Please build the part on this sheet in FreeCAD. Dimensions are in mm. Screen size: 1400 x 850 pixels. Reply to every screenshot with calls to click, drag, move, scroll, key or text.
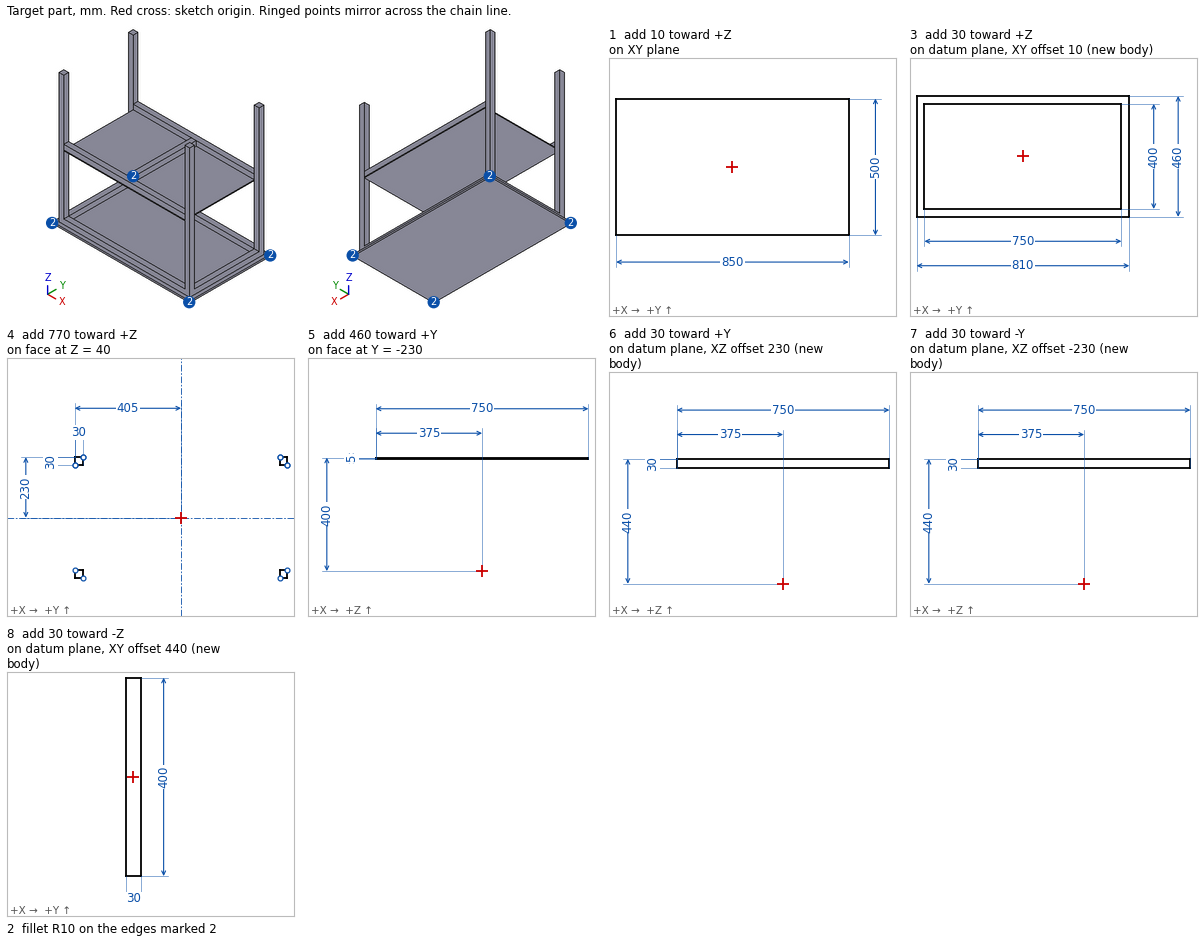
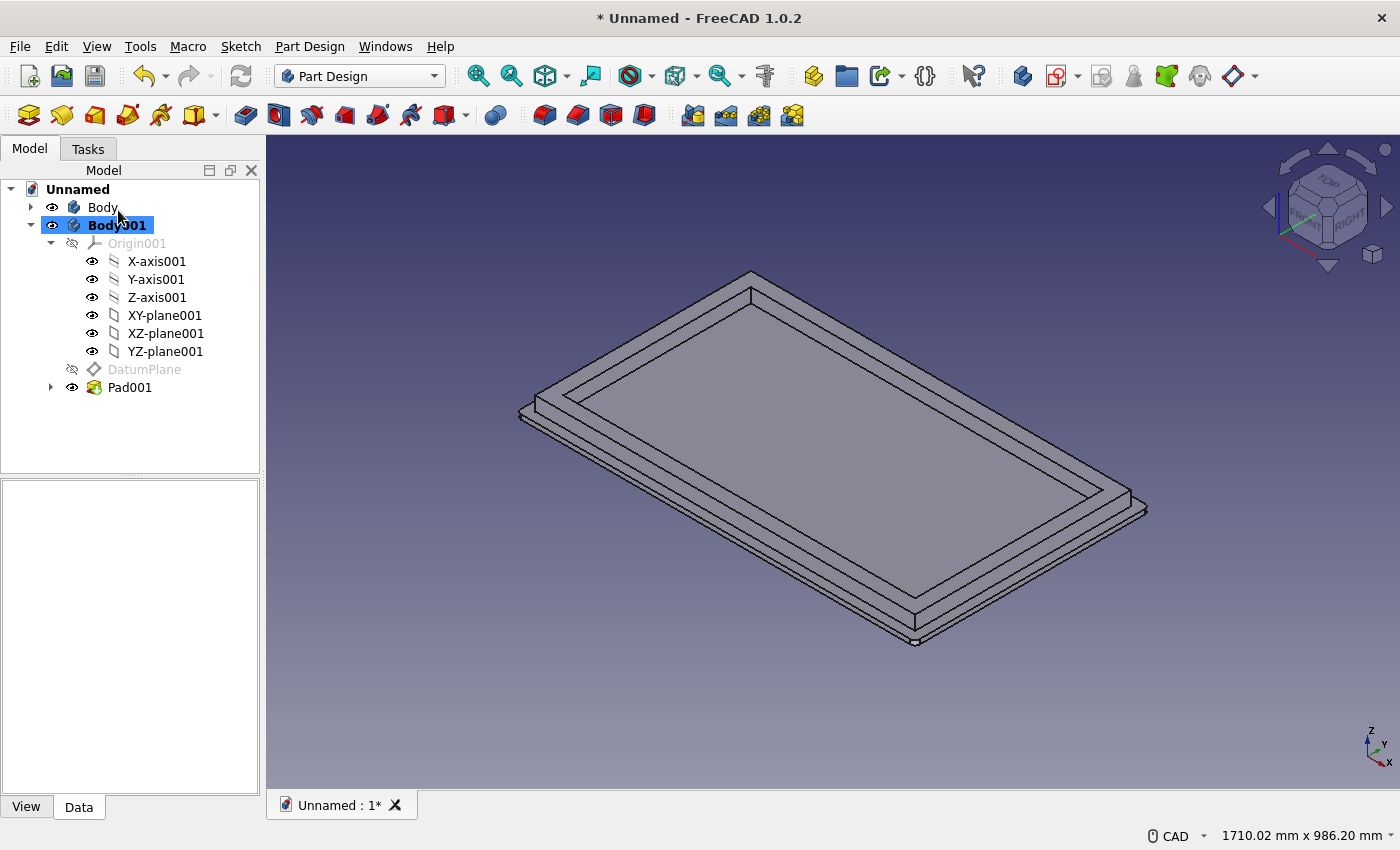
click(1049, 525)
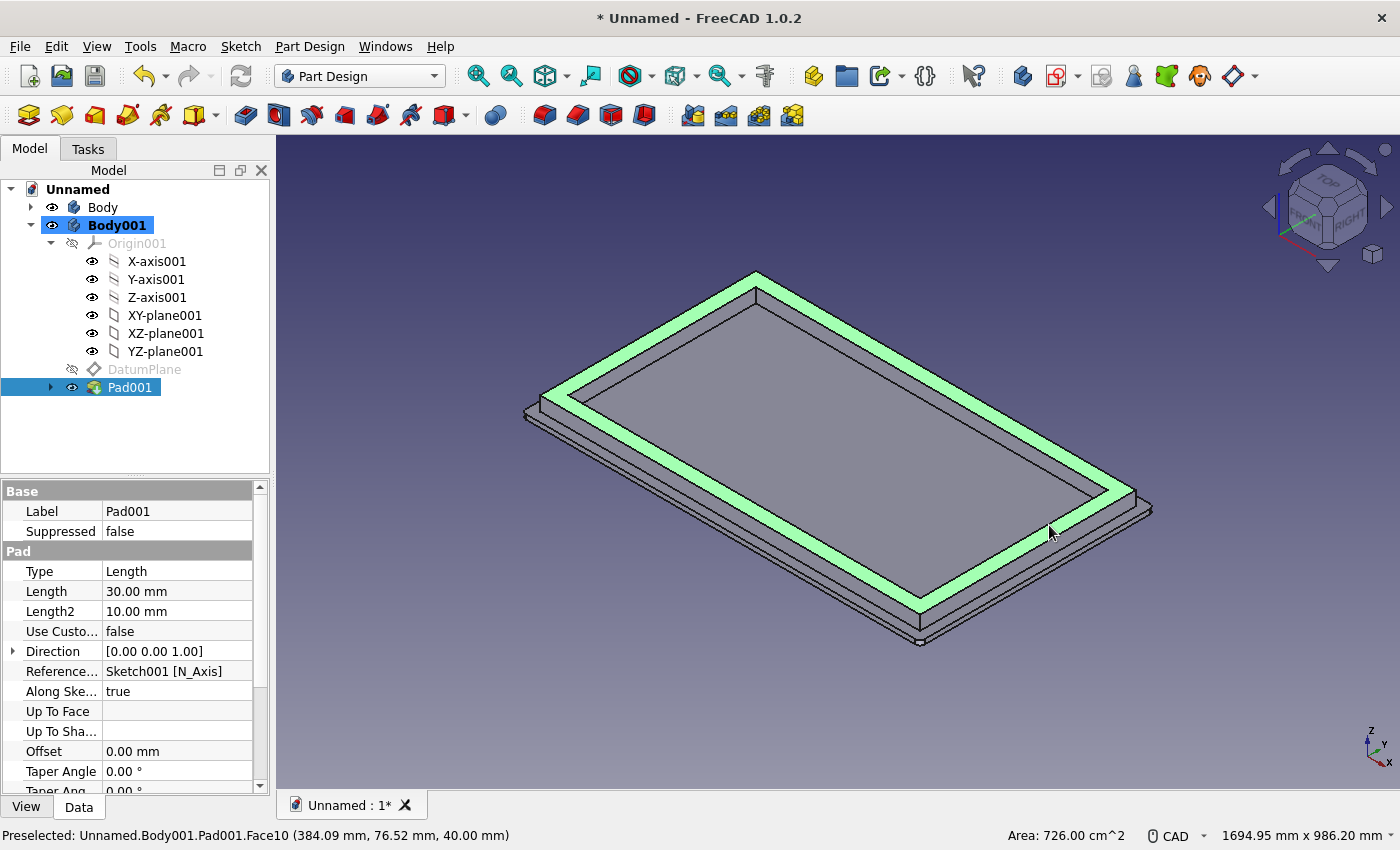
click(1056, 76)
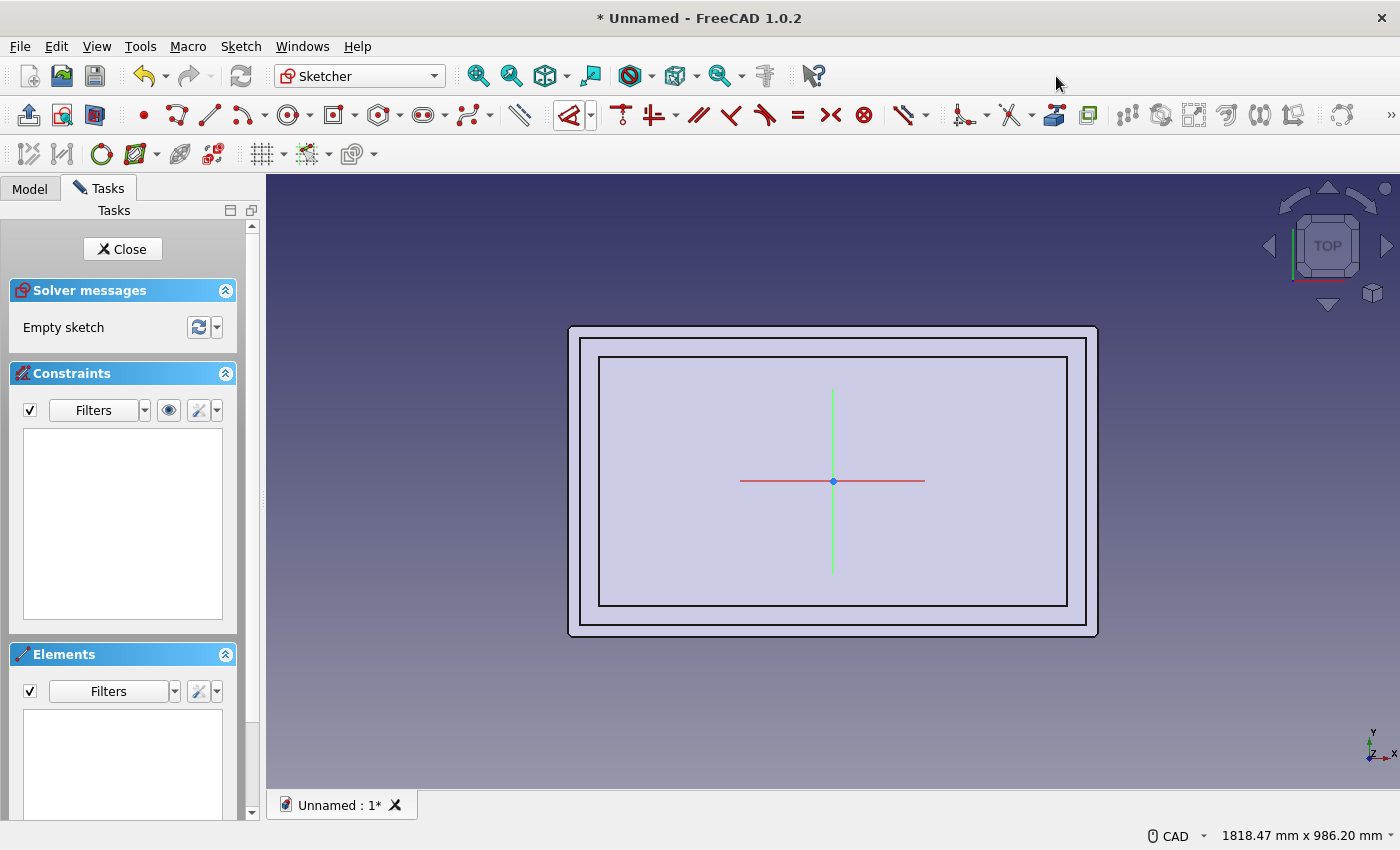
key(g)
key(r)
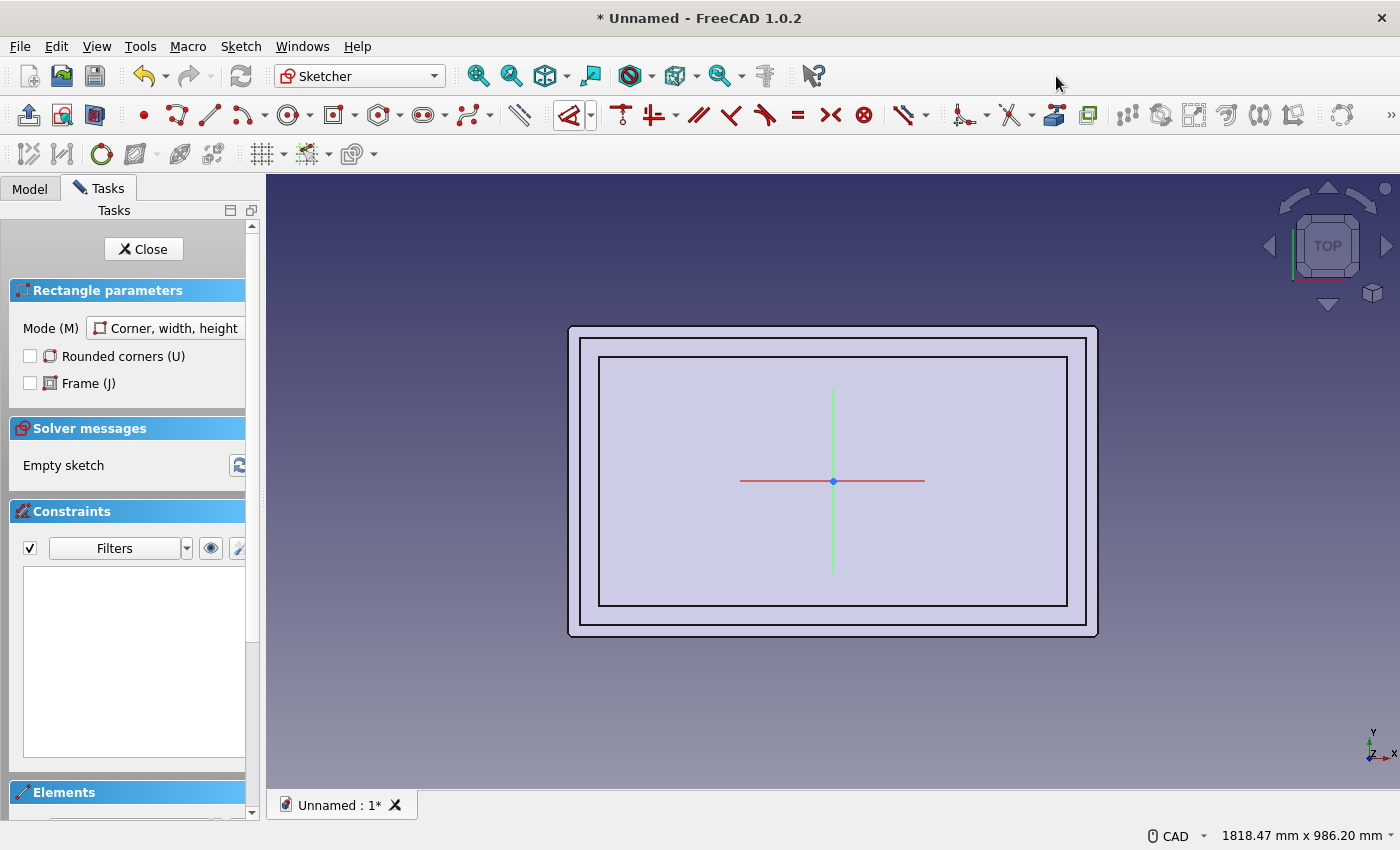
click(580, 338)
click(599, 357)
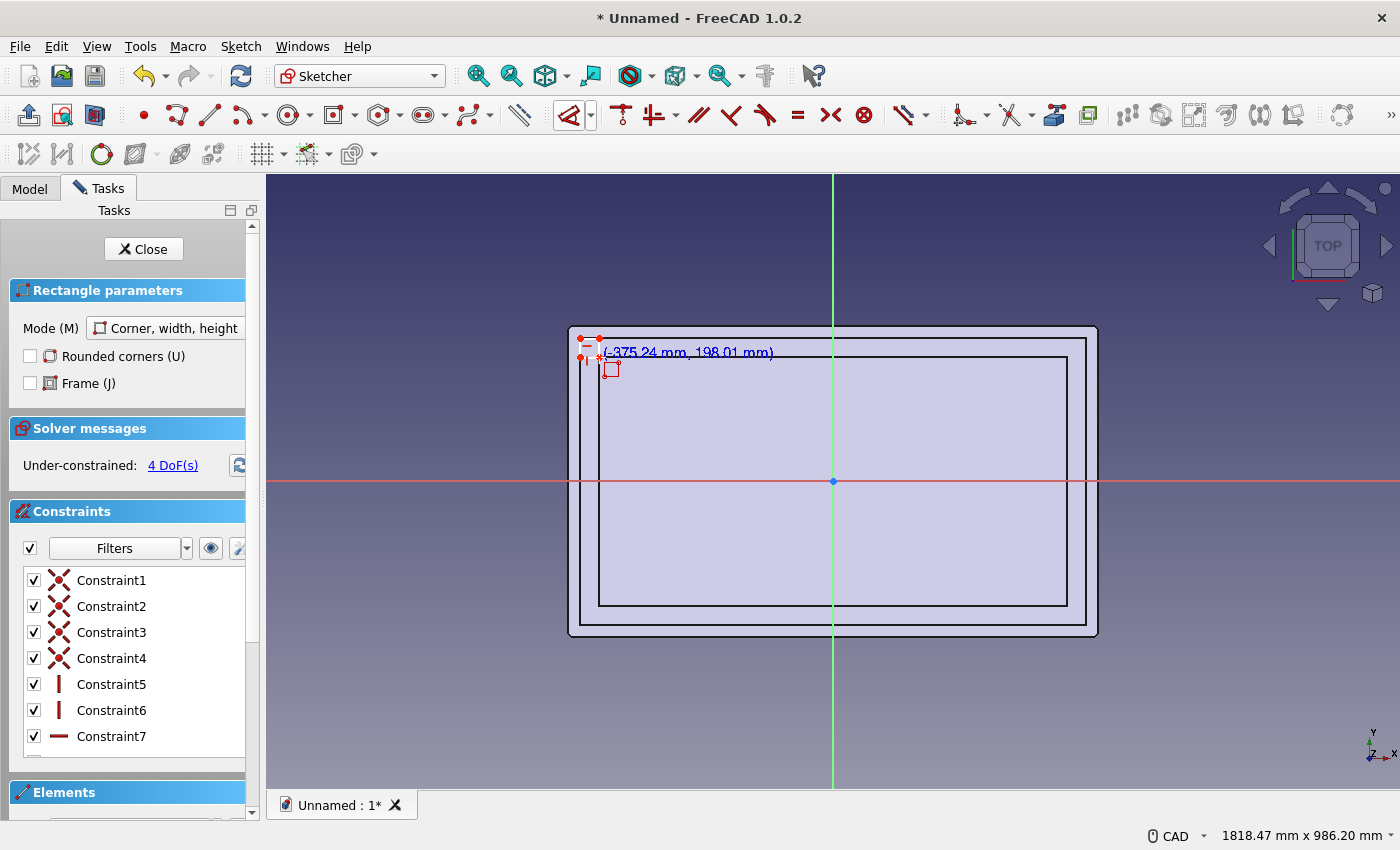
click(1067, 606)
click(1086, 625)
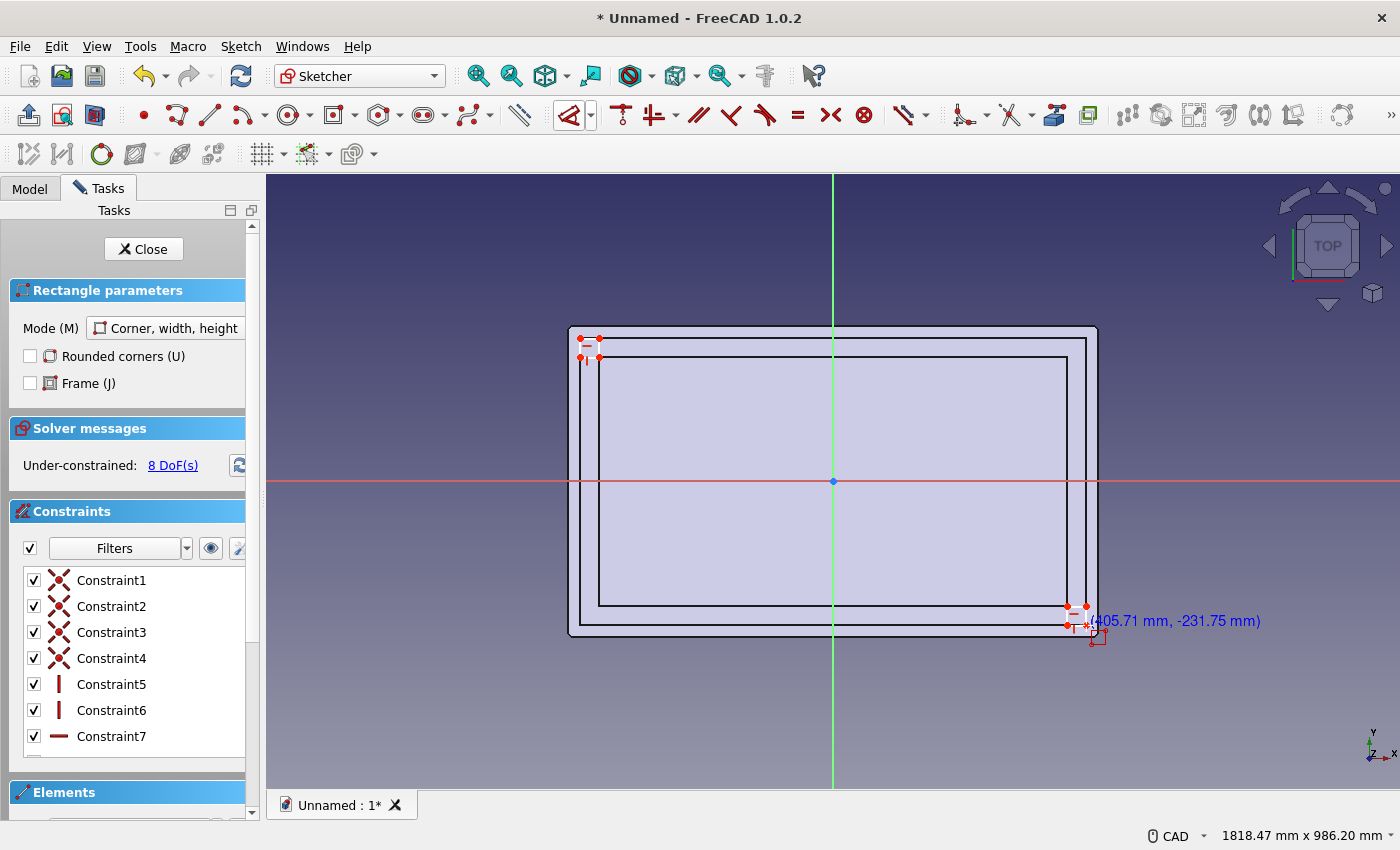
click(1067, 338)
click(1086, 357)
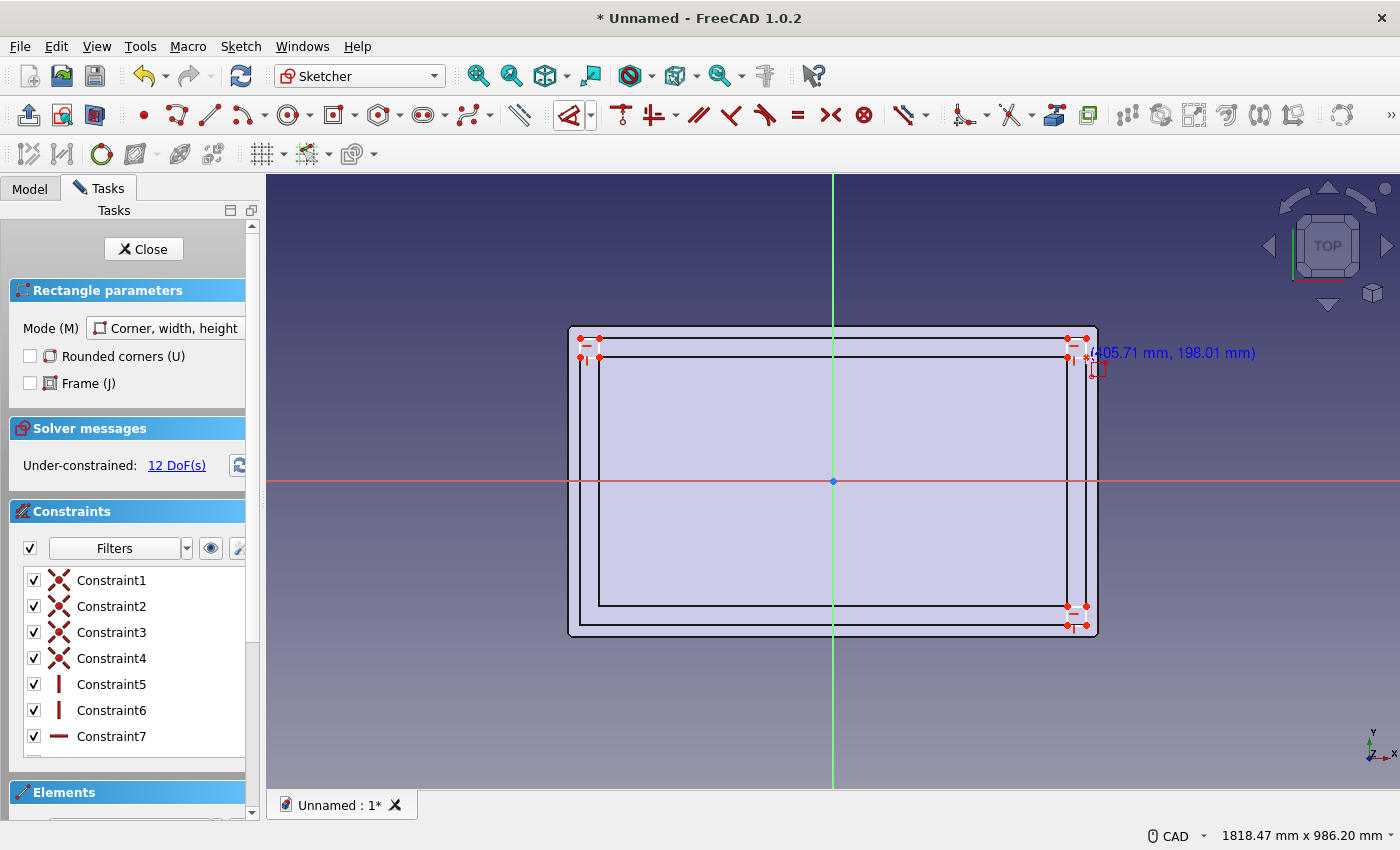
click(580, 606)
click(599, 625)
key(Escape)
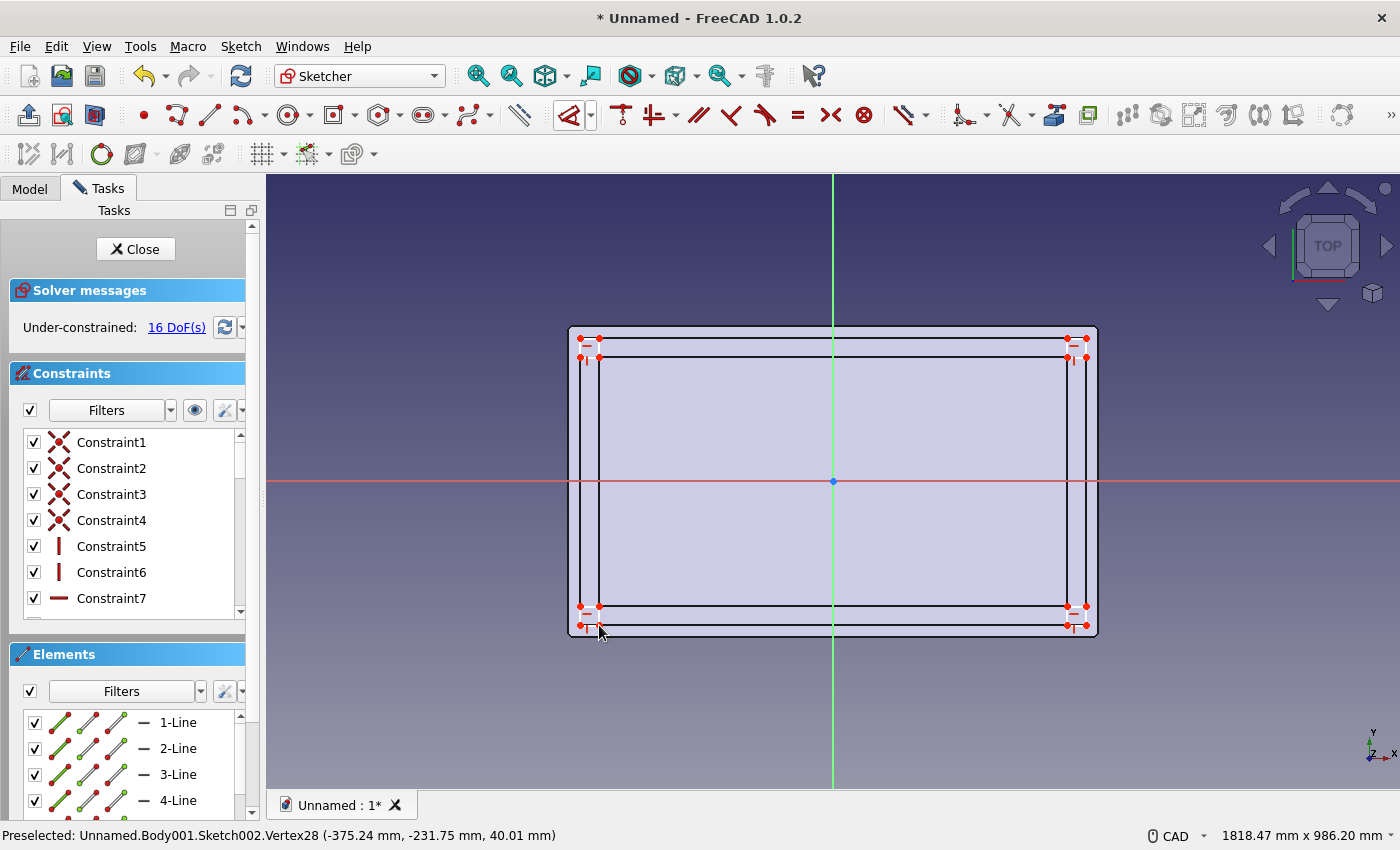
click(599, 339)